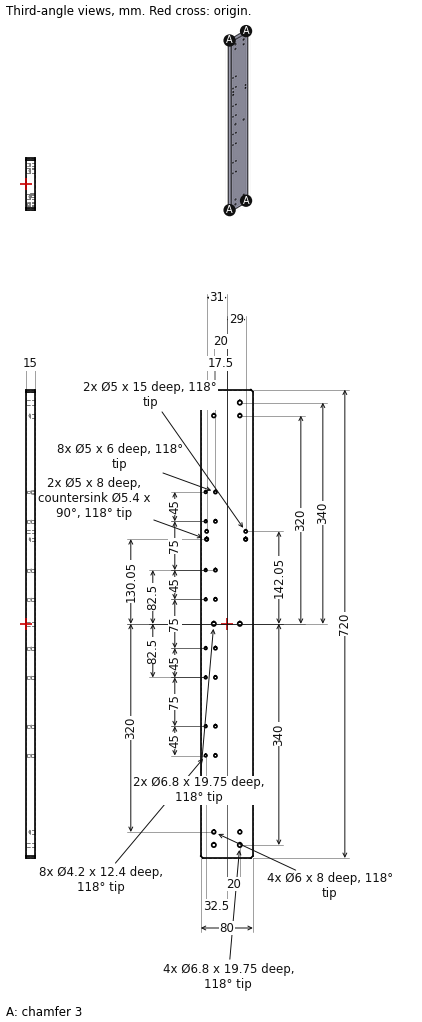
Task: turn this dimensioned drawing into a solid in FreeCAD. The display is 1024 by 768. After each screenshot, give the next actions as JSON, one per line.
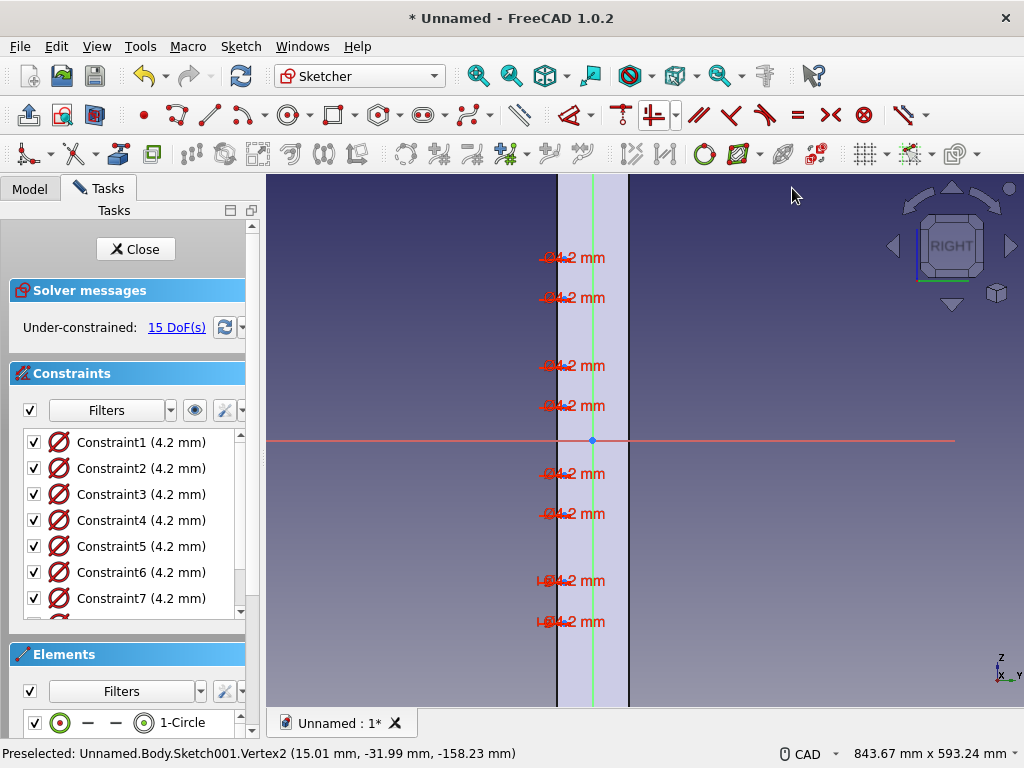
{"action": "left_click", "coordinate": [564, 583]}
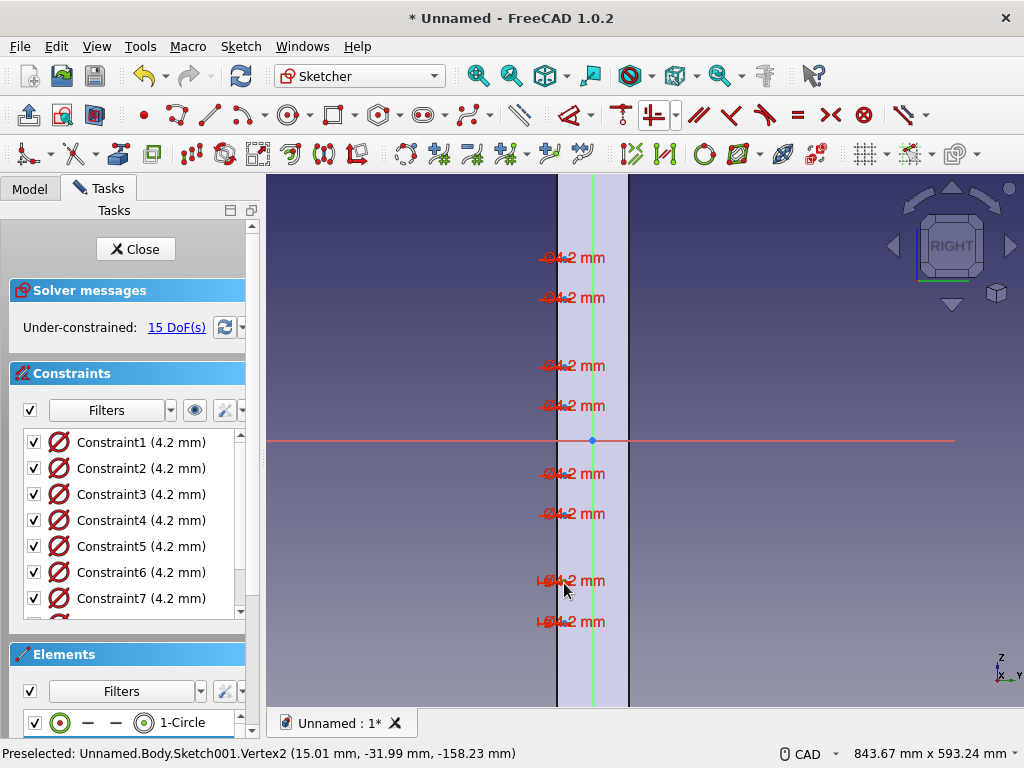
{"action": "left_click", "coordinate": [564, 516]}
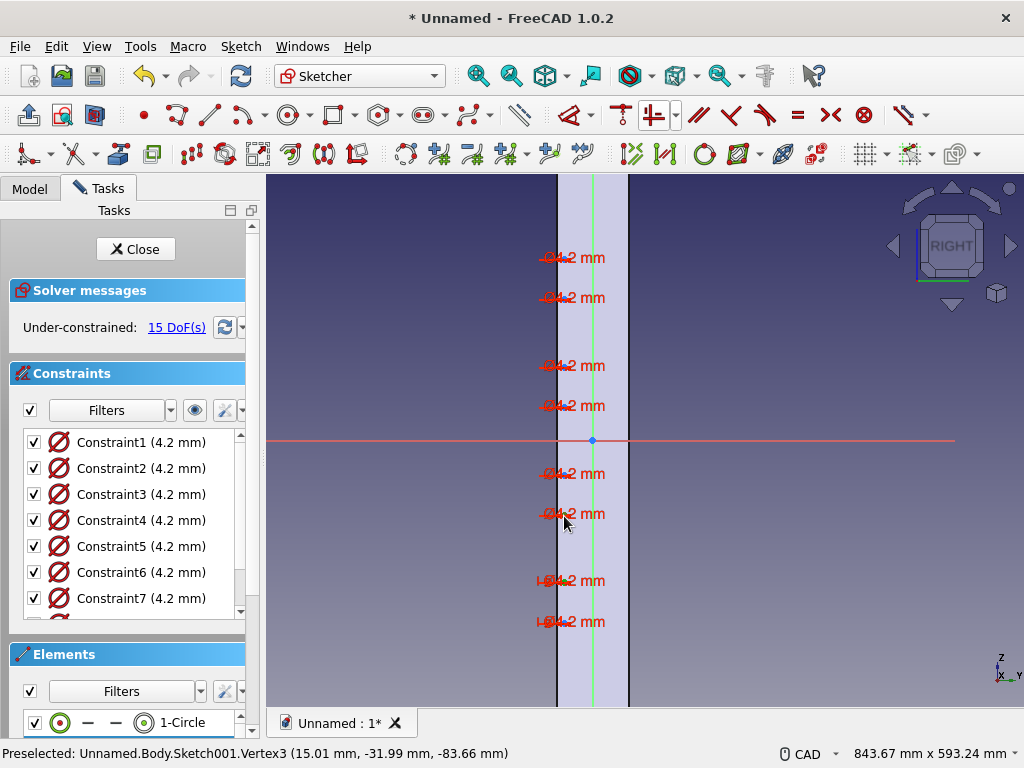
{"action": "key", "text": "v"}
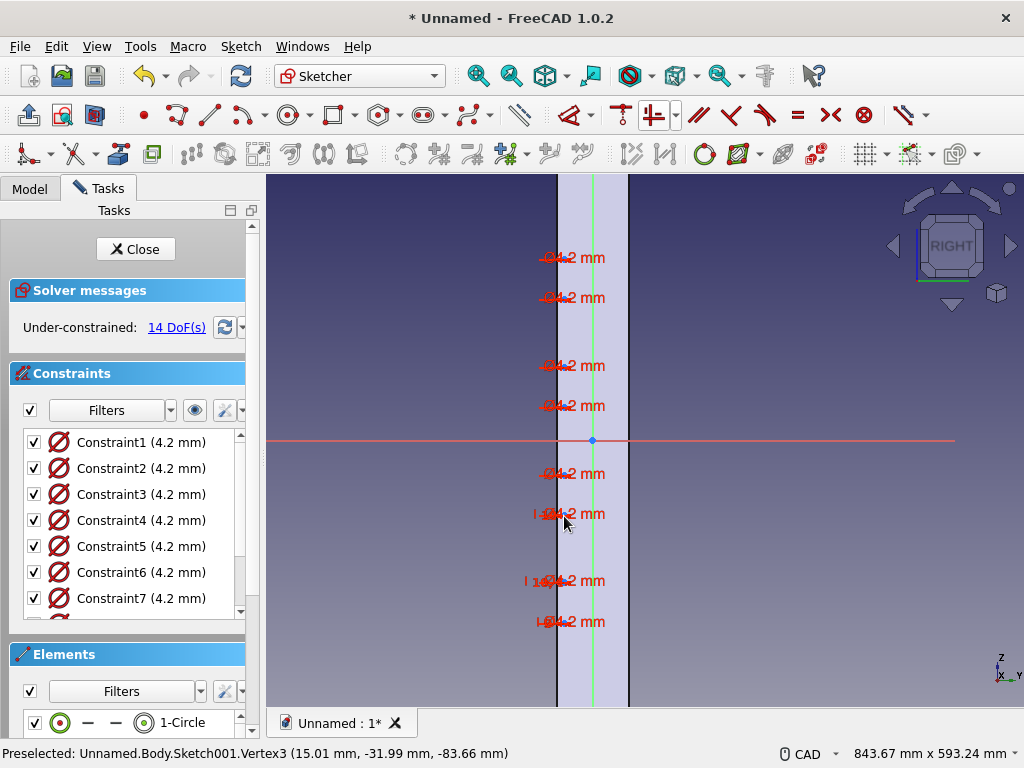
{"action": "left_click", "coordinate": [564, 516]}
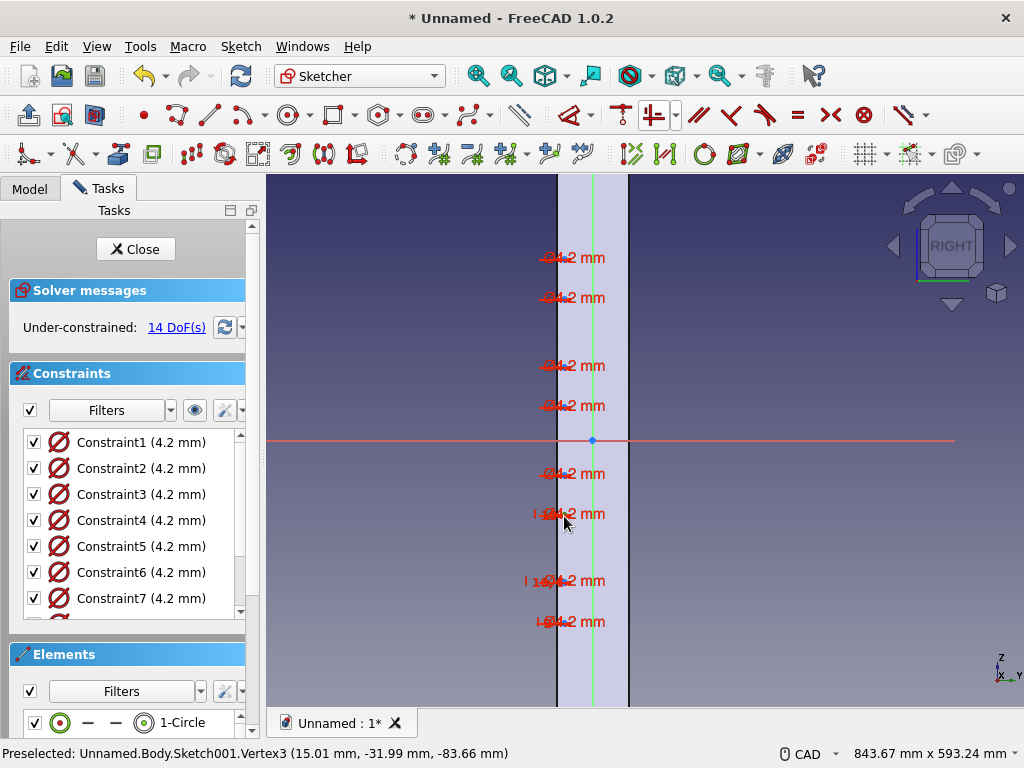
{"action": "left_click", "coordinate": [564, 476]}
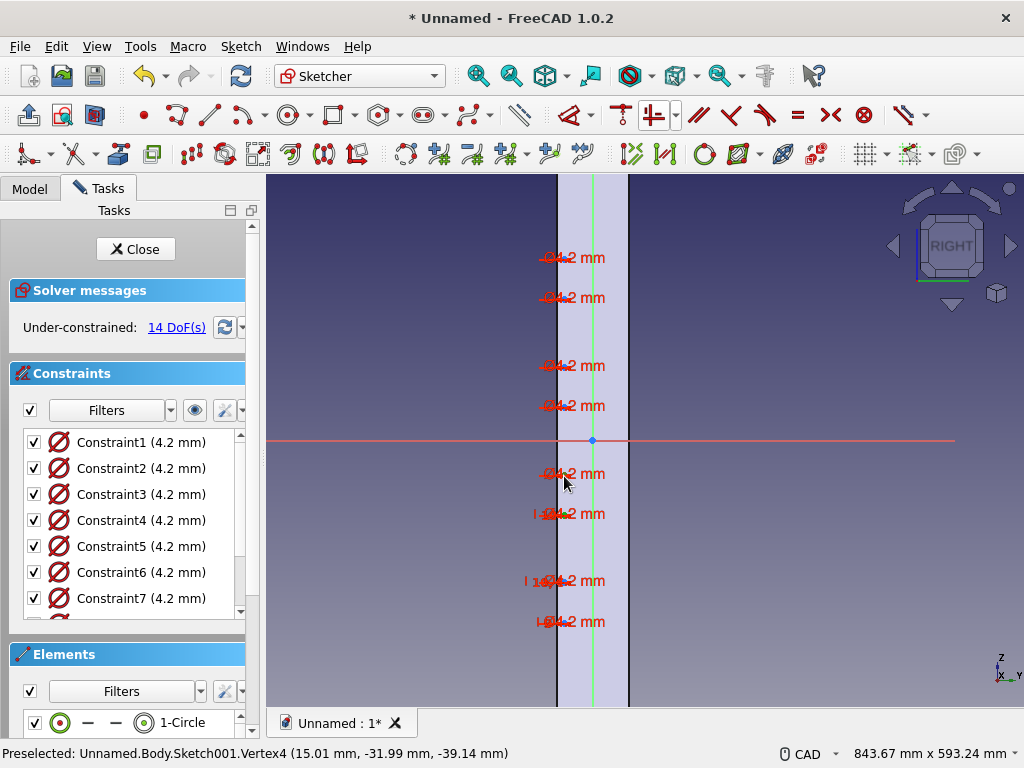
{"action": "key", "text": "v"}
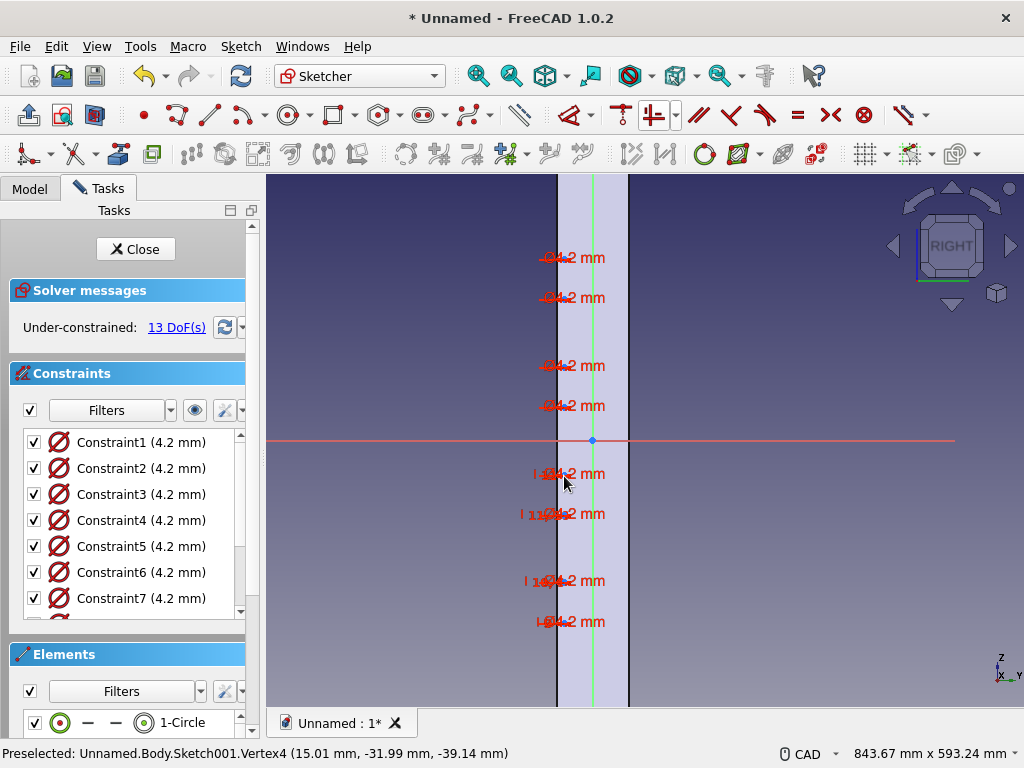
{"action": "left_click", "coordinate": [564, 476]}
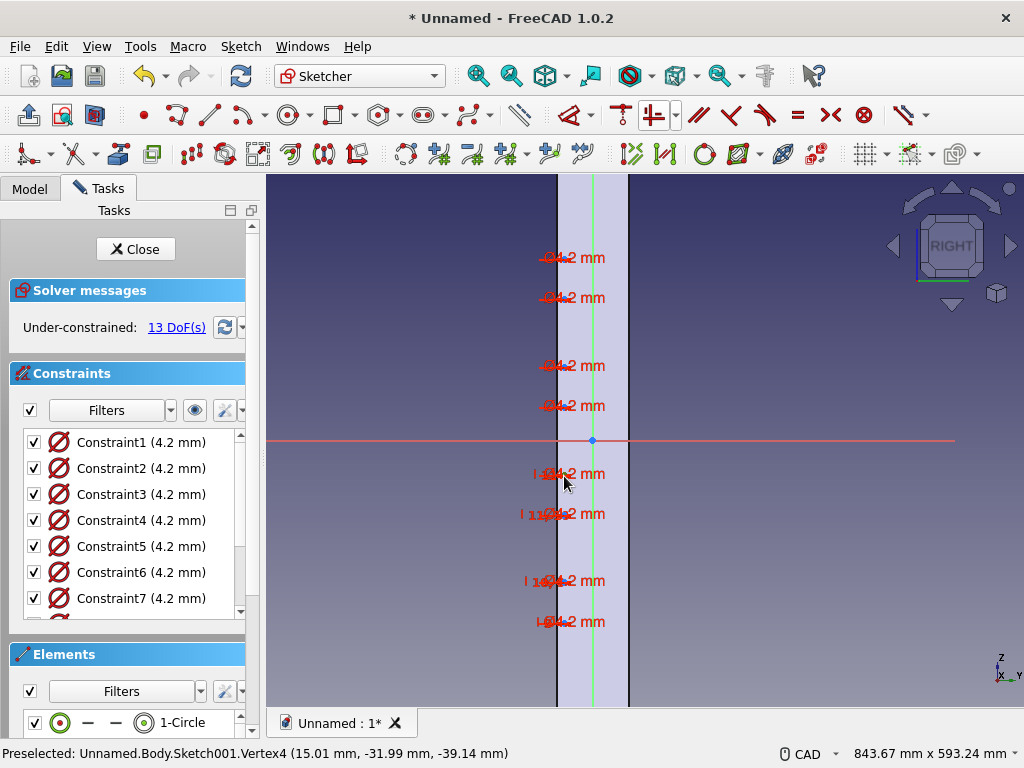
{"action": "left_click", "coordinate": [564, 408]}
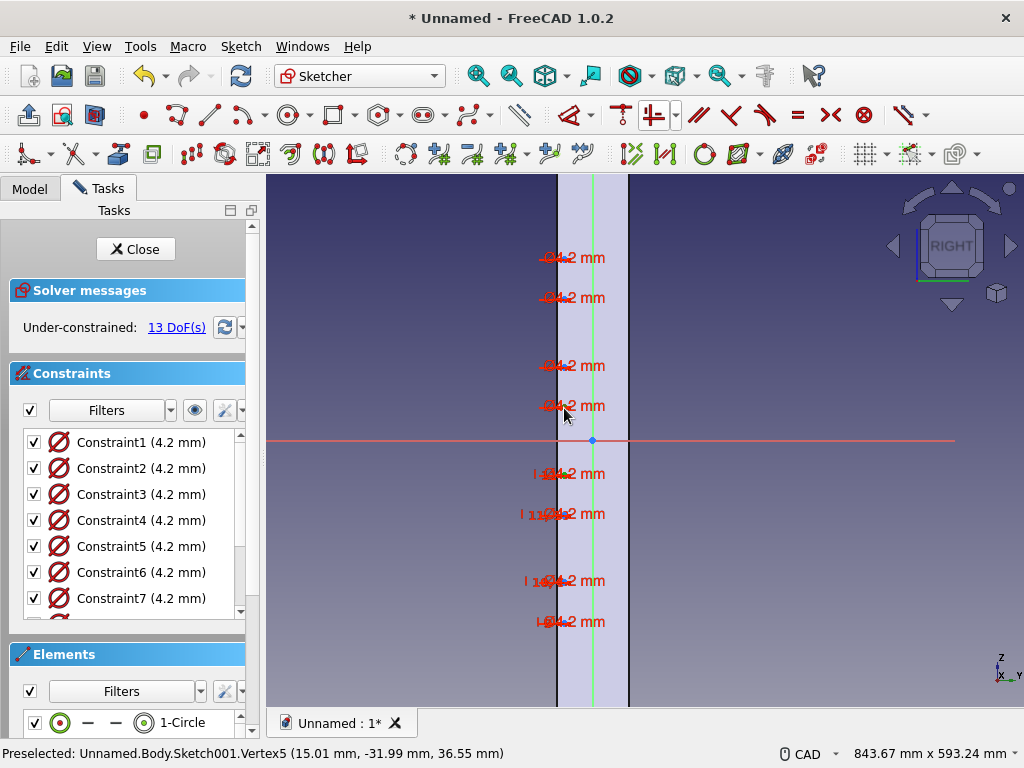
{"action": "key", "text": "v"}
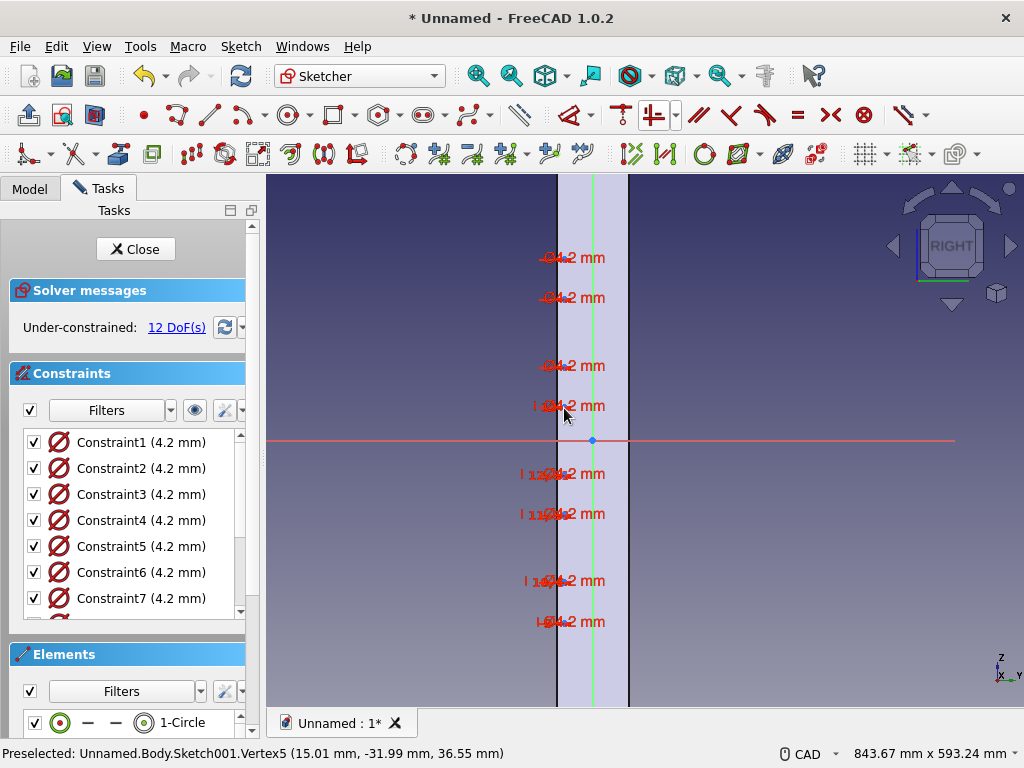
{"action": "left_click", "coordinate": [564, 408]}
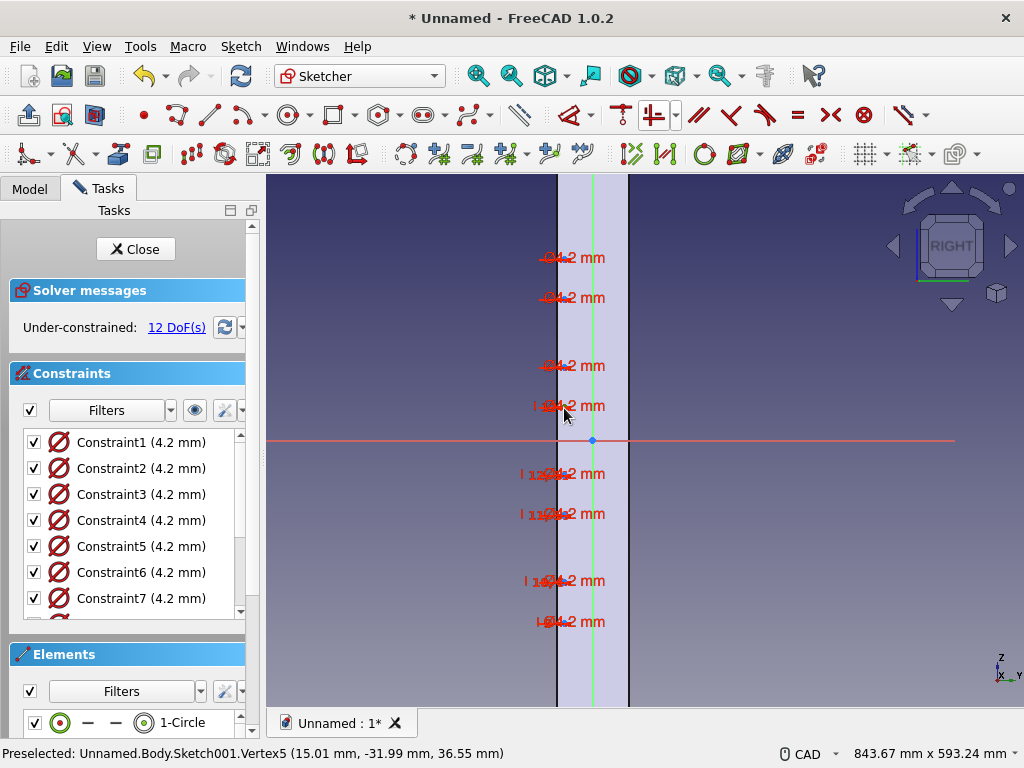
{"action": "left_click", "coordinate": [564, 368]}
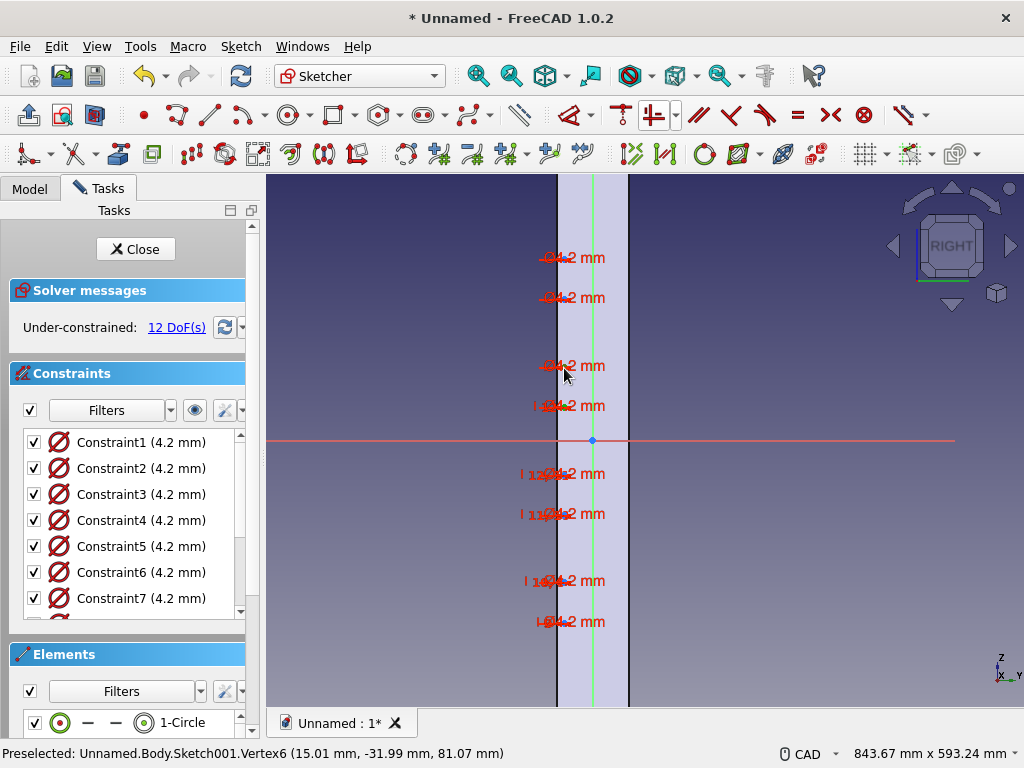
{"action": "key", "text": "v"}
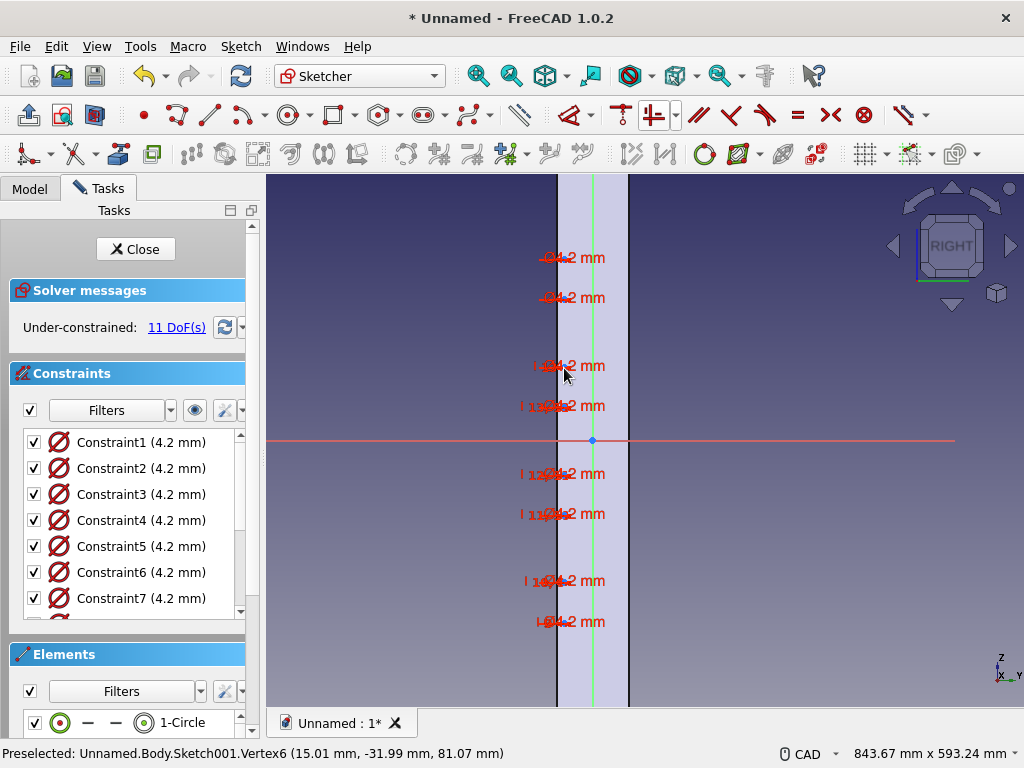
{"action": "left_click", "coordinate": [564, 368]}